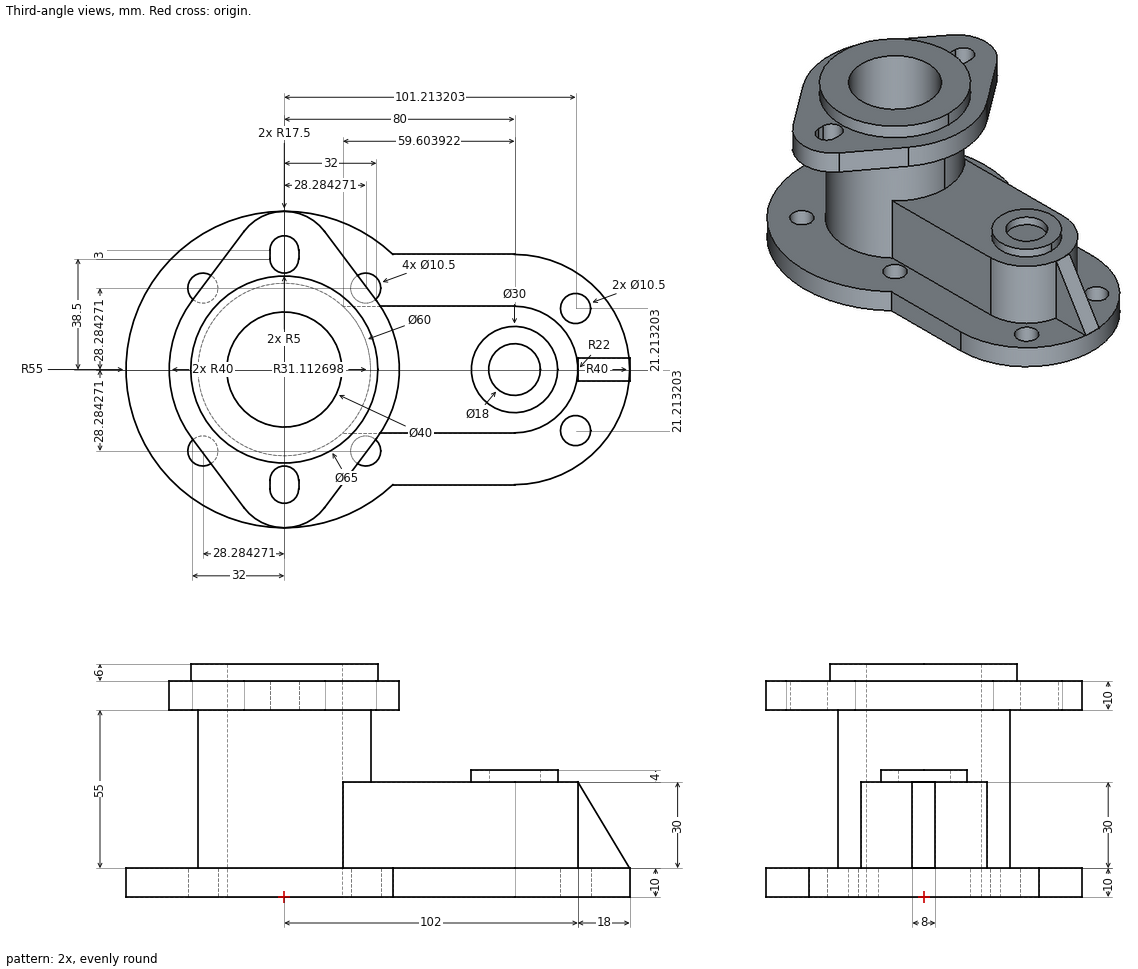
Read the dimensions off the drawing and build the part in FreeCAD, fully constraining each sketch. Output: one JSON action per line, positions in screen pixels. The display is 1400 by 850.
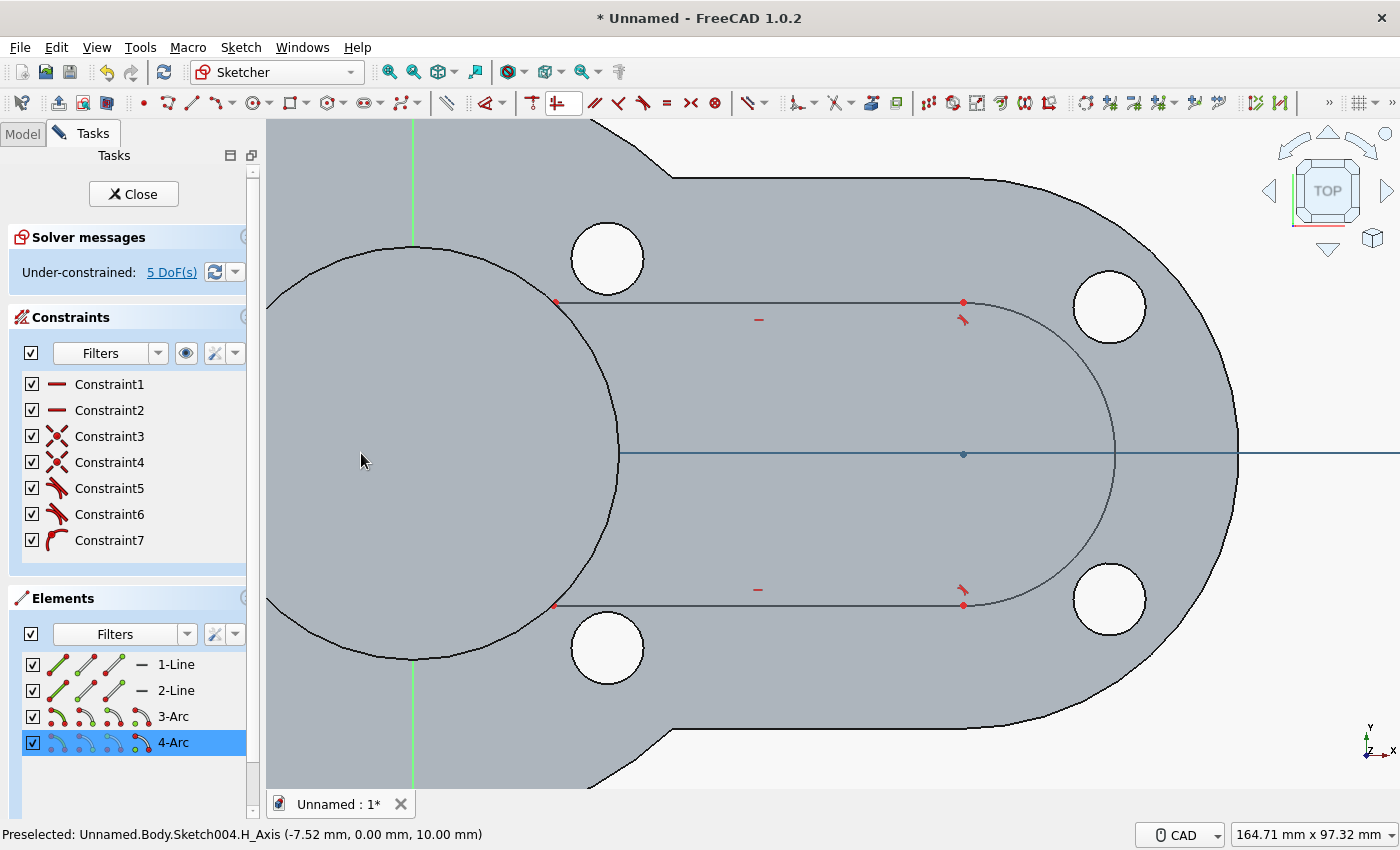
{"action": "key", "text": "c"}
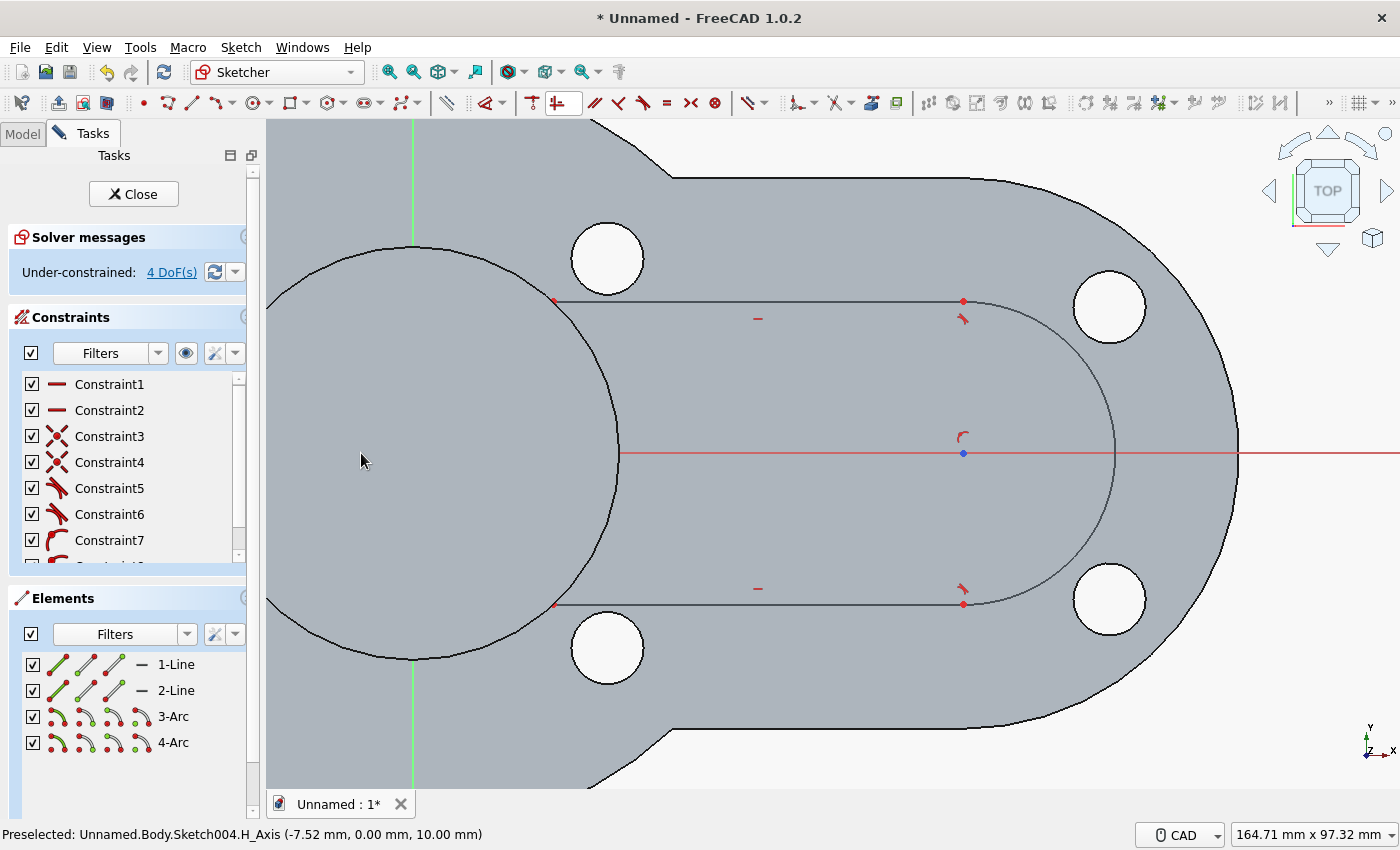
{"action": "key", "text": "d"}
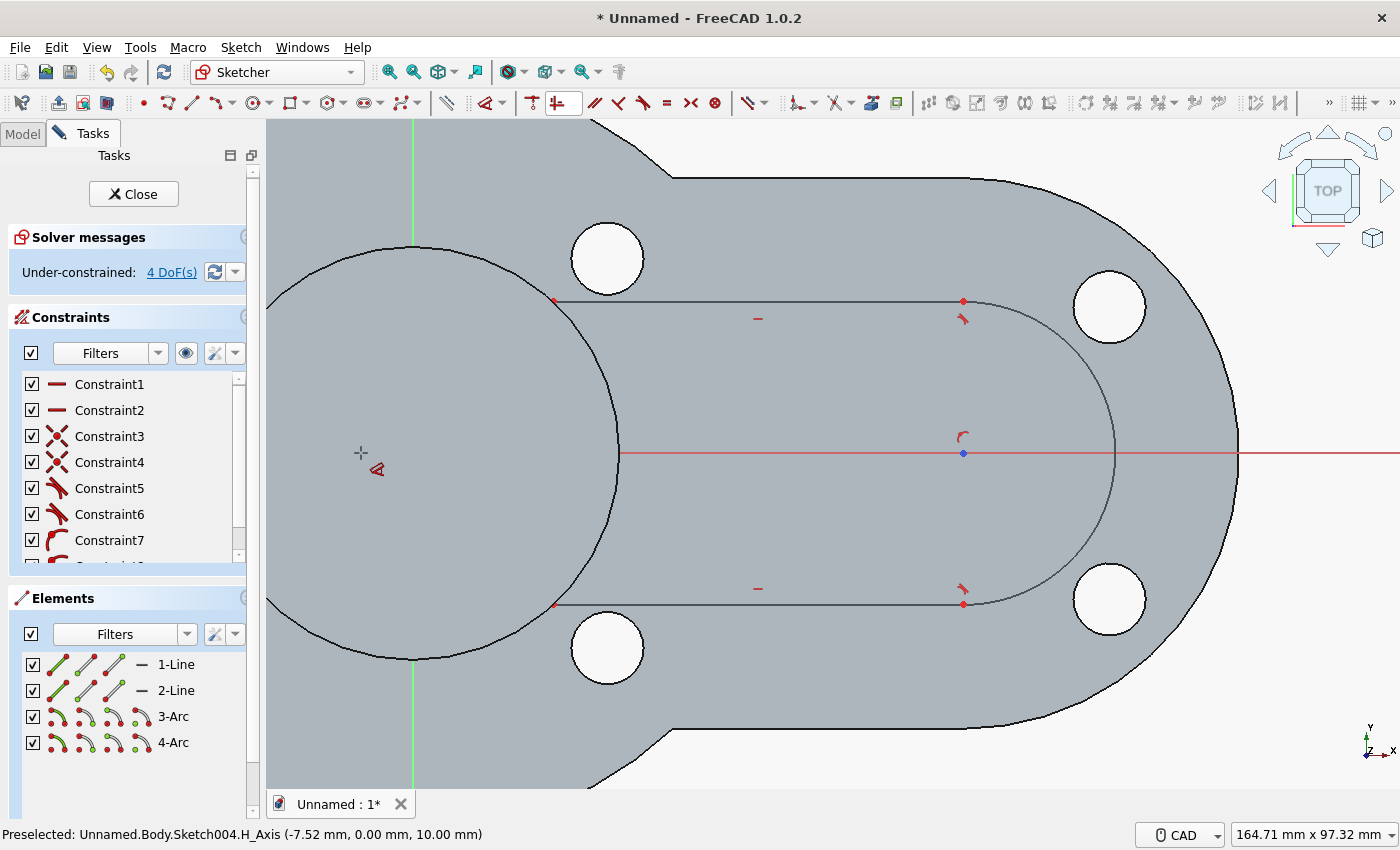
{"action": "left_click", "coordinate": [605, 520]}
{"action": "left_click", "coordinate": [635, 530]}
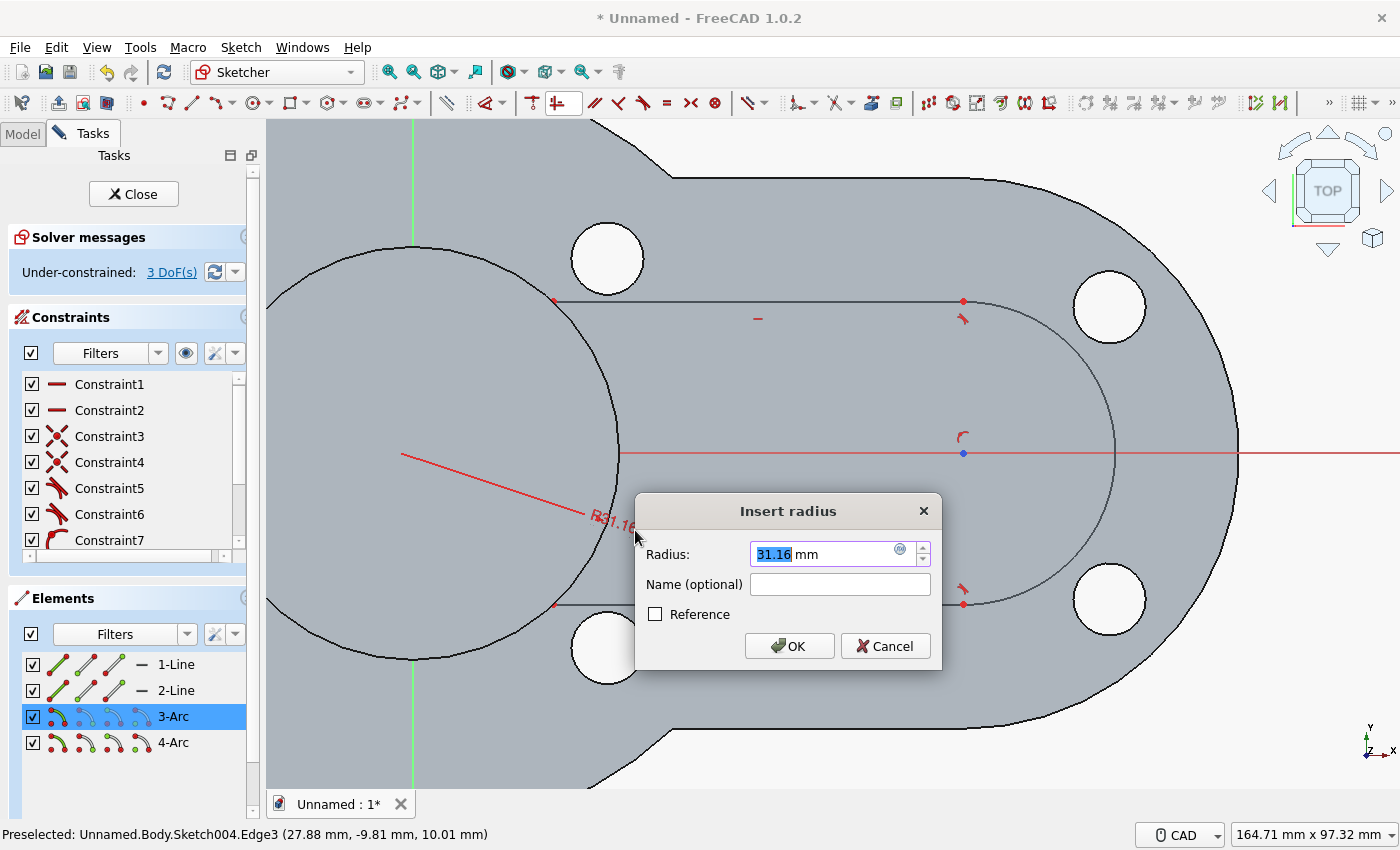
{"action": "type", "text": "31.112698"}
{"action": "key", "text": "Return"}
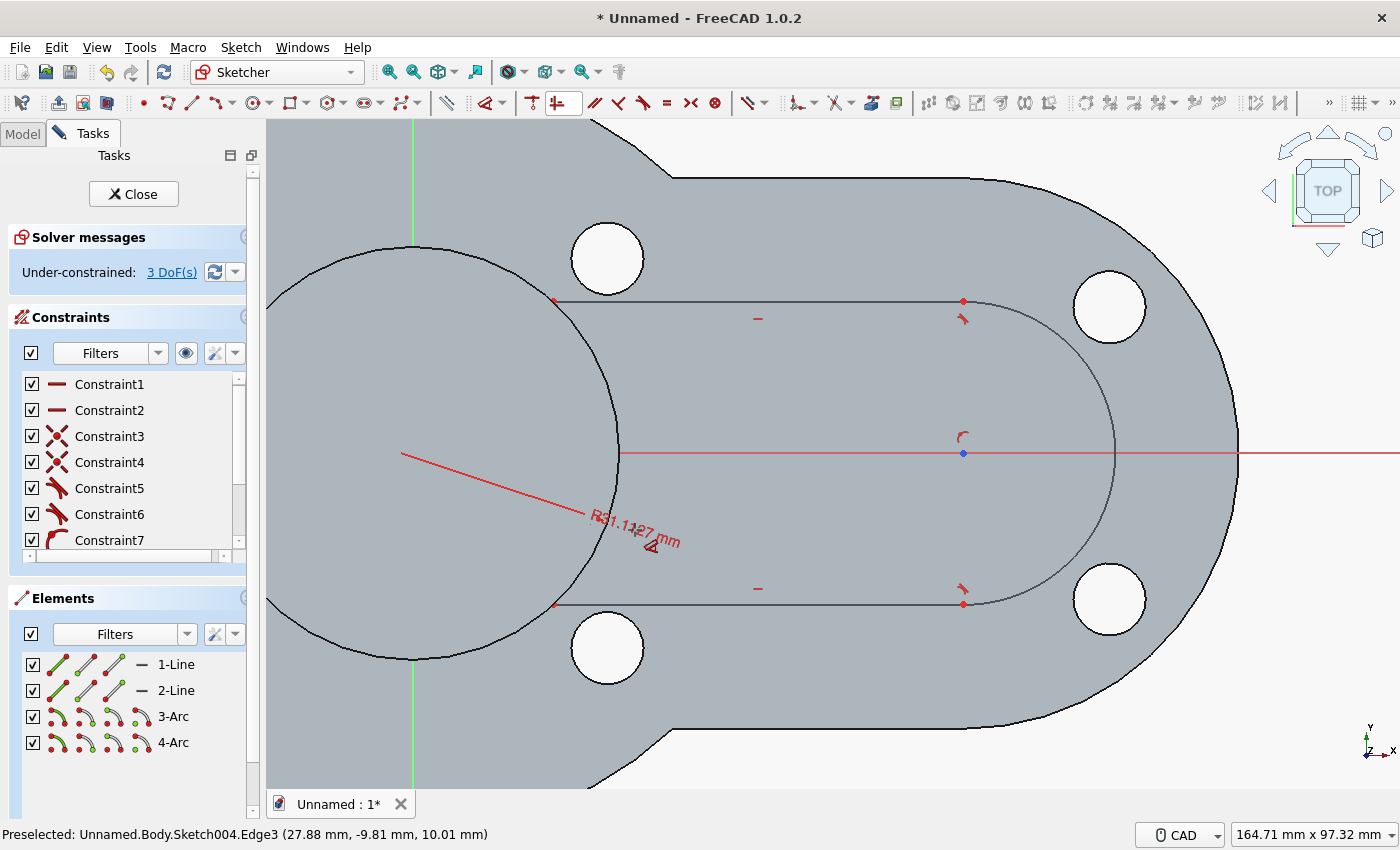
{"action": "left_click", "coordinate": [1086, 542]}
{"action": "left_click", "coordinate": [1112, 561]}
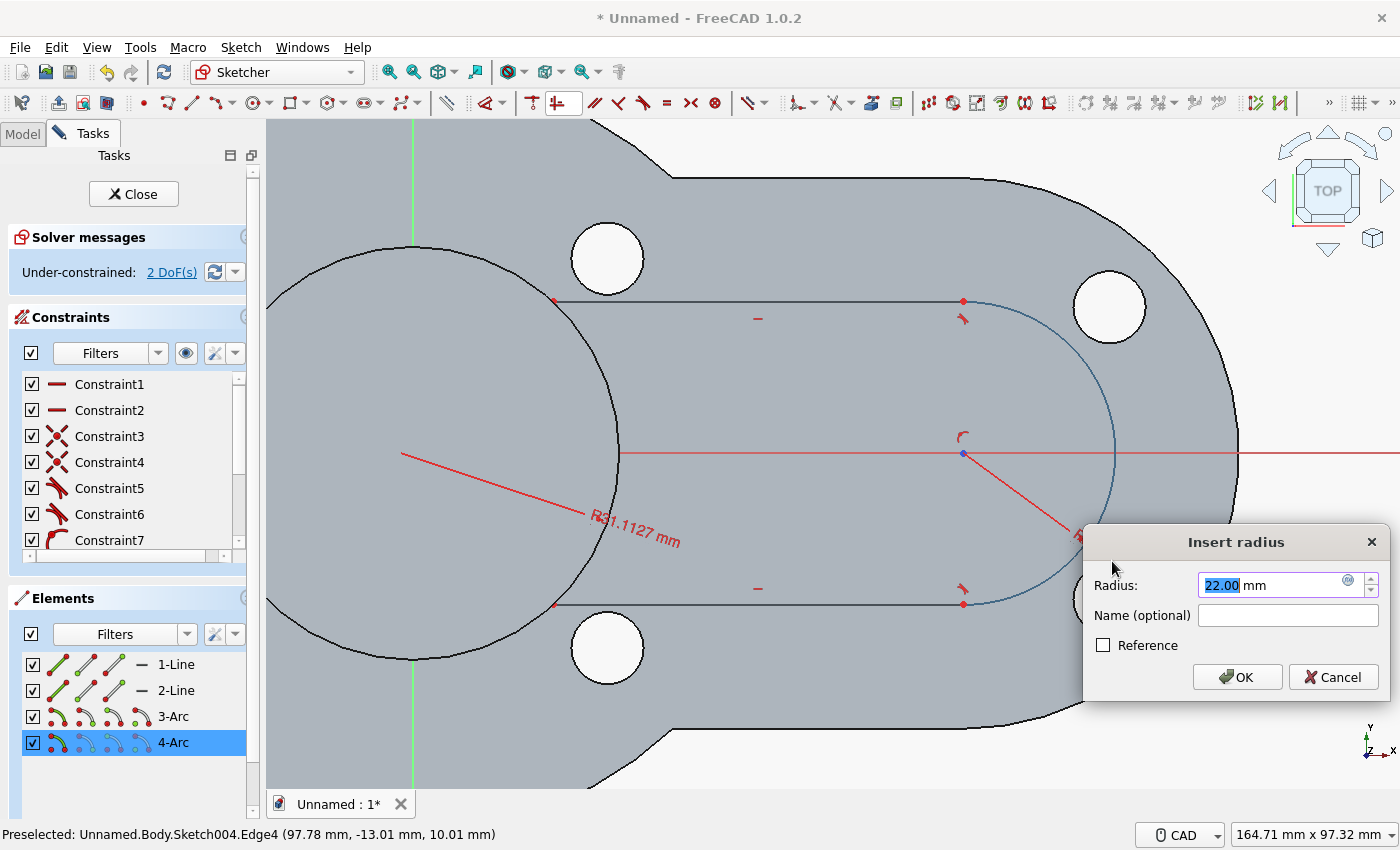
{"action": "type", "text": "22"}
{"action": "key", "text": "Return"}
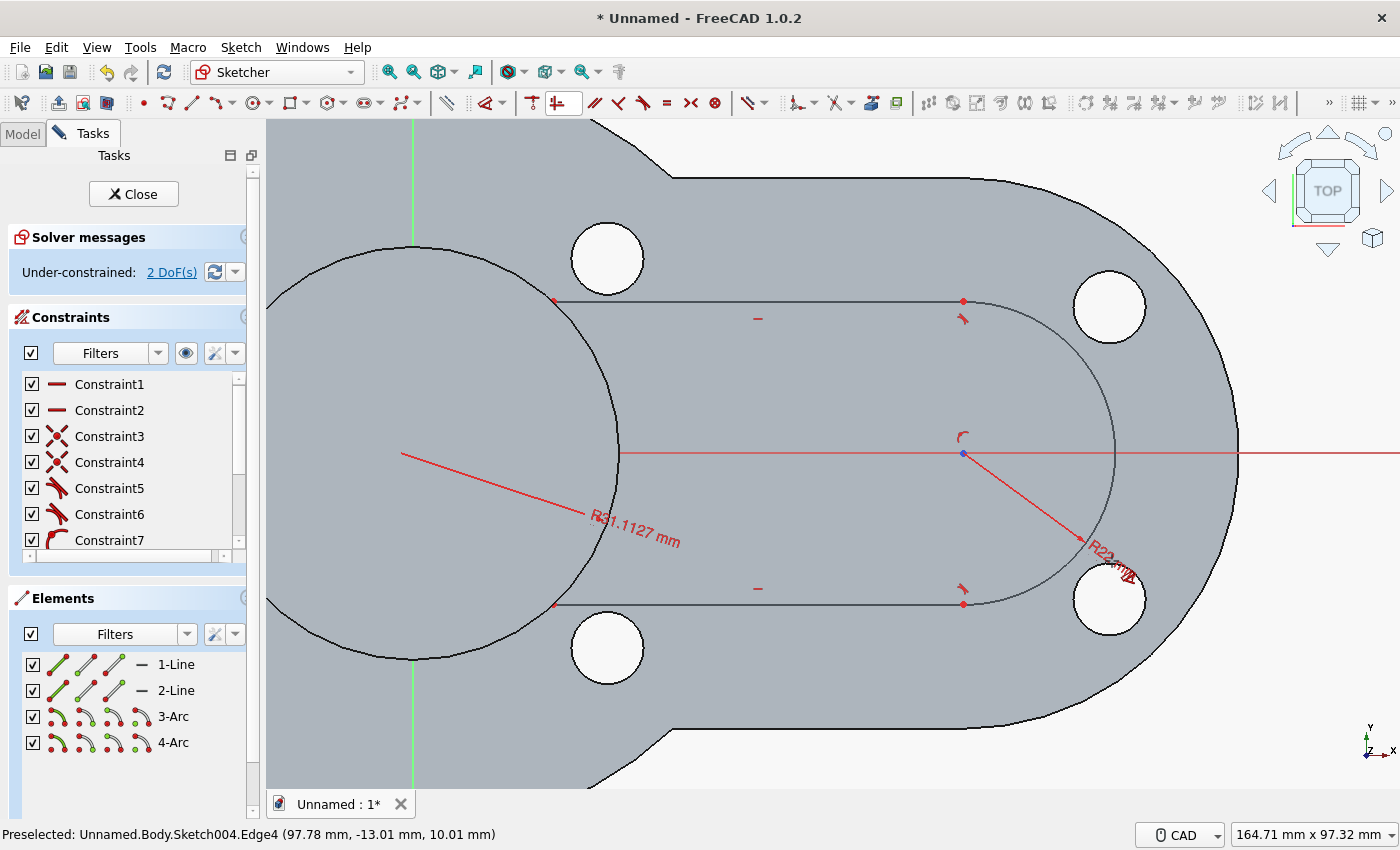
{"action": "left_click", "coordinate": [964, 302]}
{"action": "left_click", "coordinate": [688, 268]}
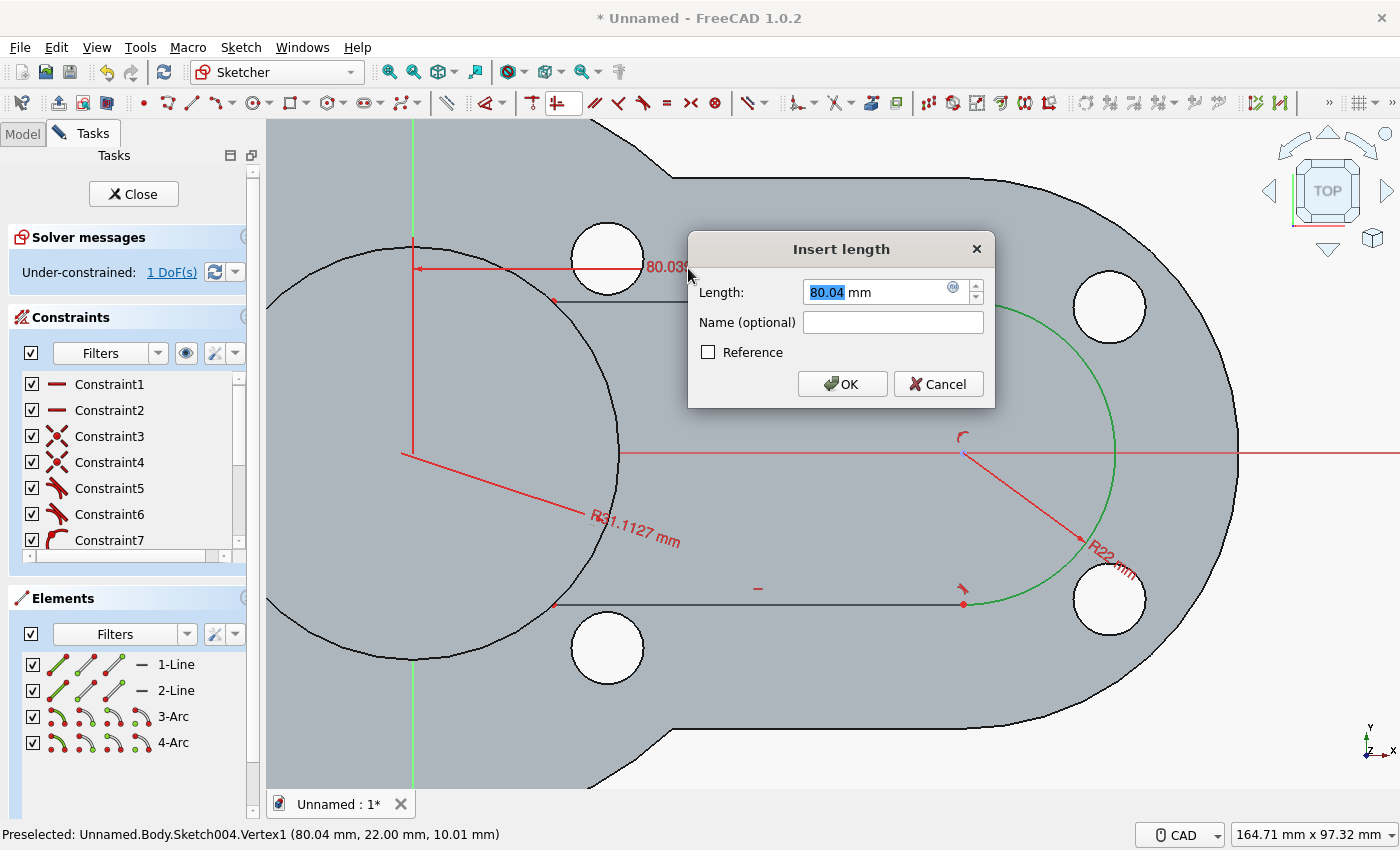
{"action": "type", "text": "80"}
{"action": "key", "text": "Return"}